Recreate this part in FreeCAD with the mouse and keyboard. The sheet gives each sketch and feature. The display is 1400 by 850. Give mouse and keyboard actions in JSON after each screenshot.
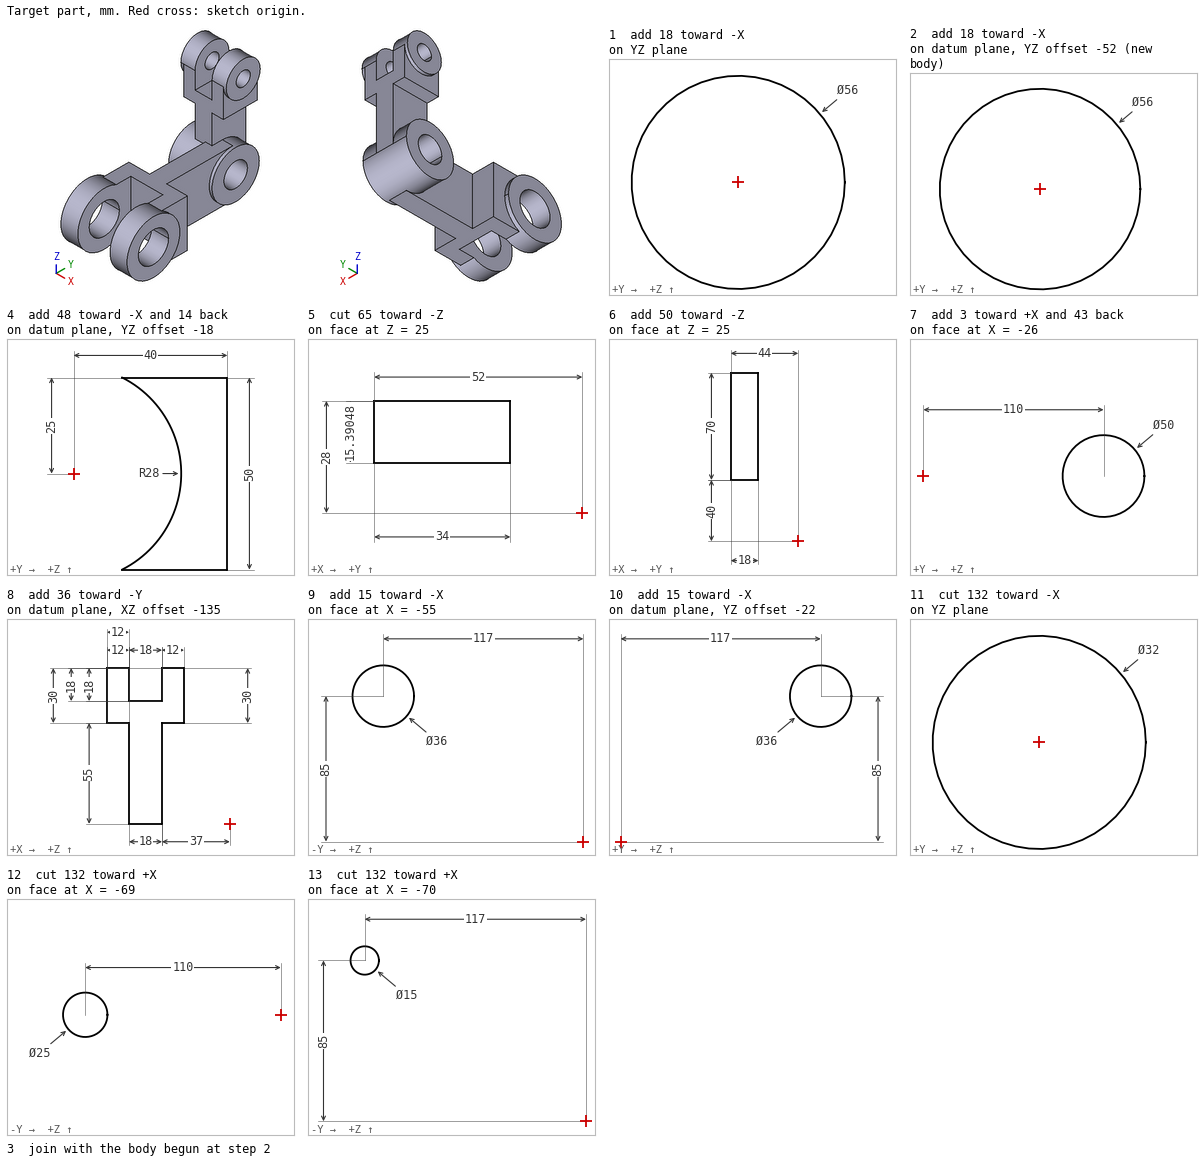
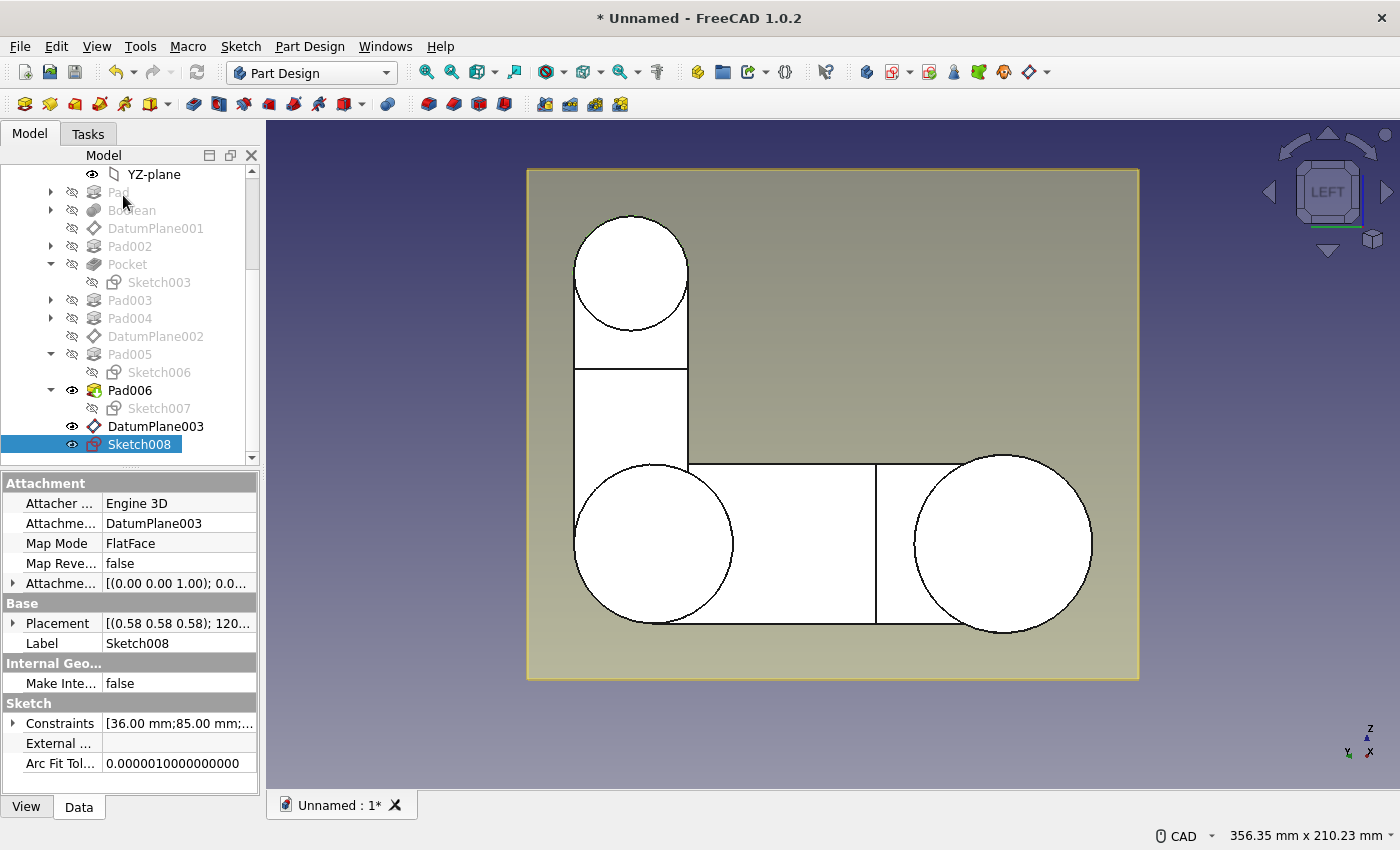
{"action": "left_click", "coordinate": [25, 104]}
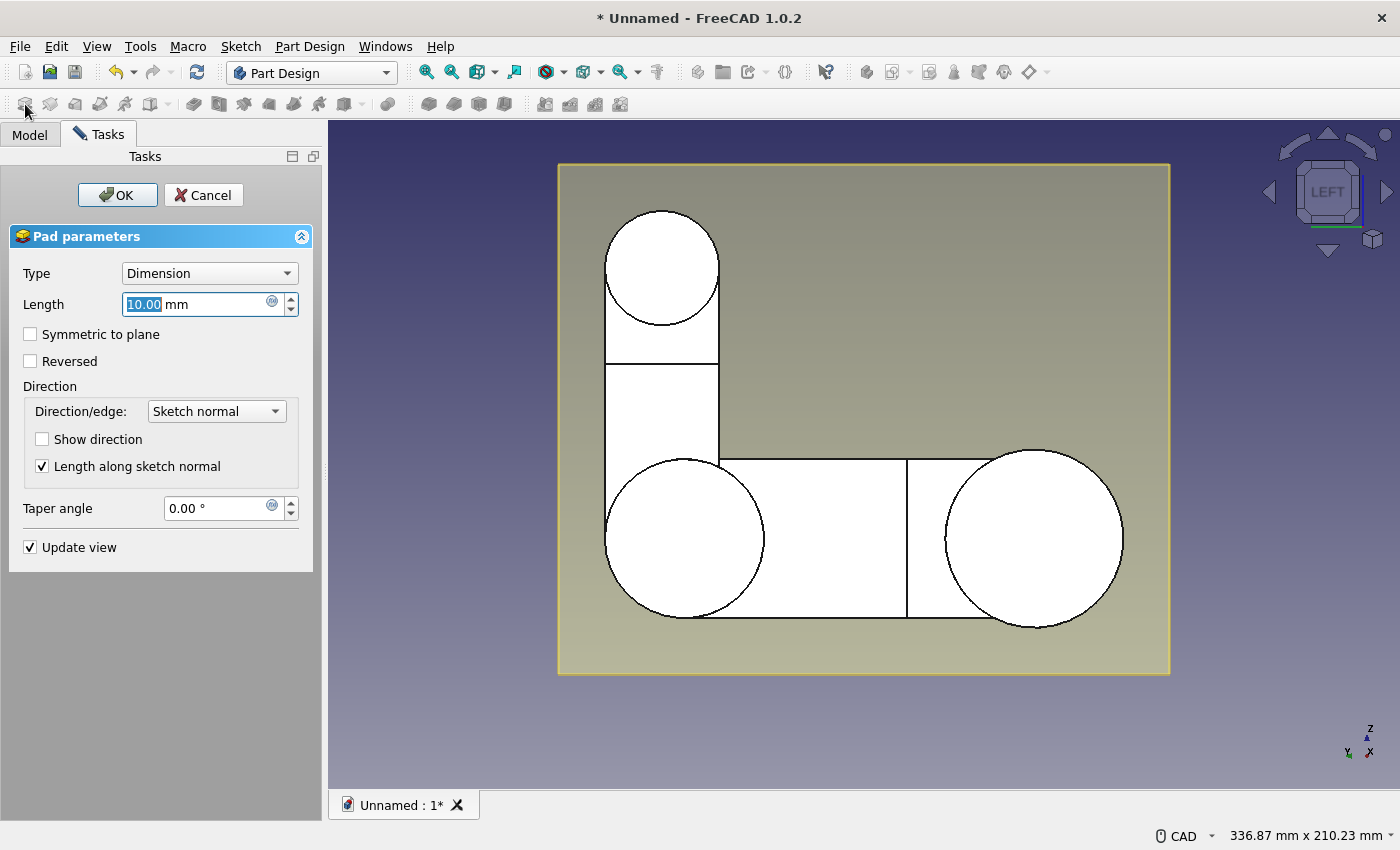
{"action": "type", "text": "15"}
{"action": "key", "text": "Tab"}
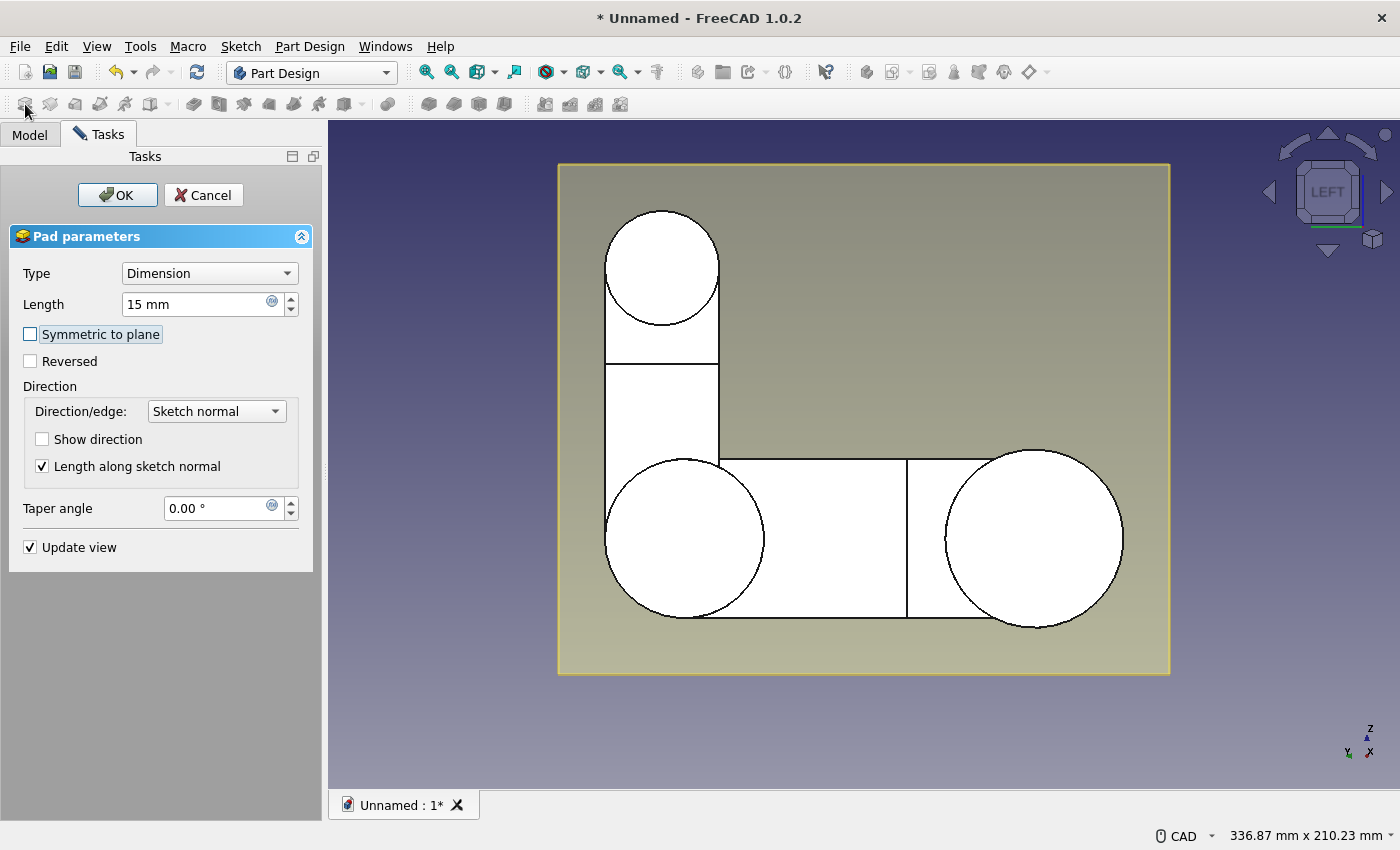
{"action": "left_click", "coordinate": [31, 361]}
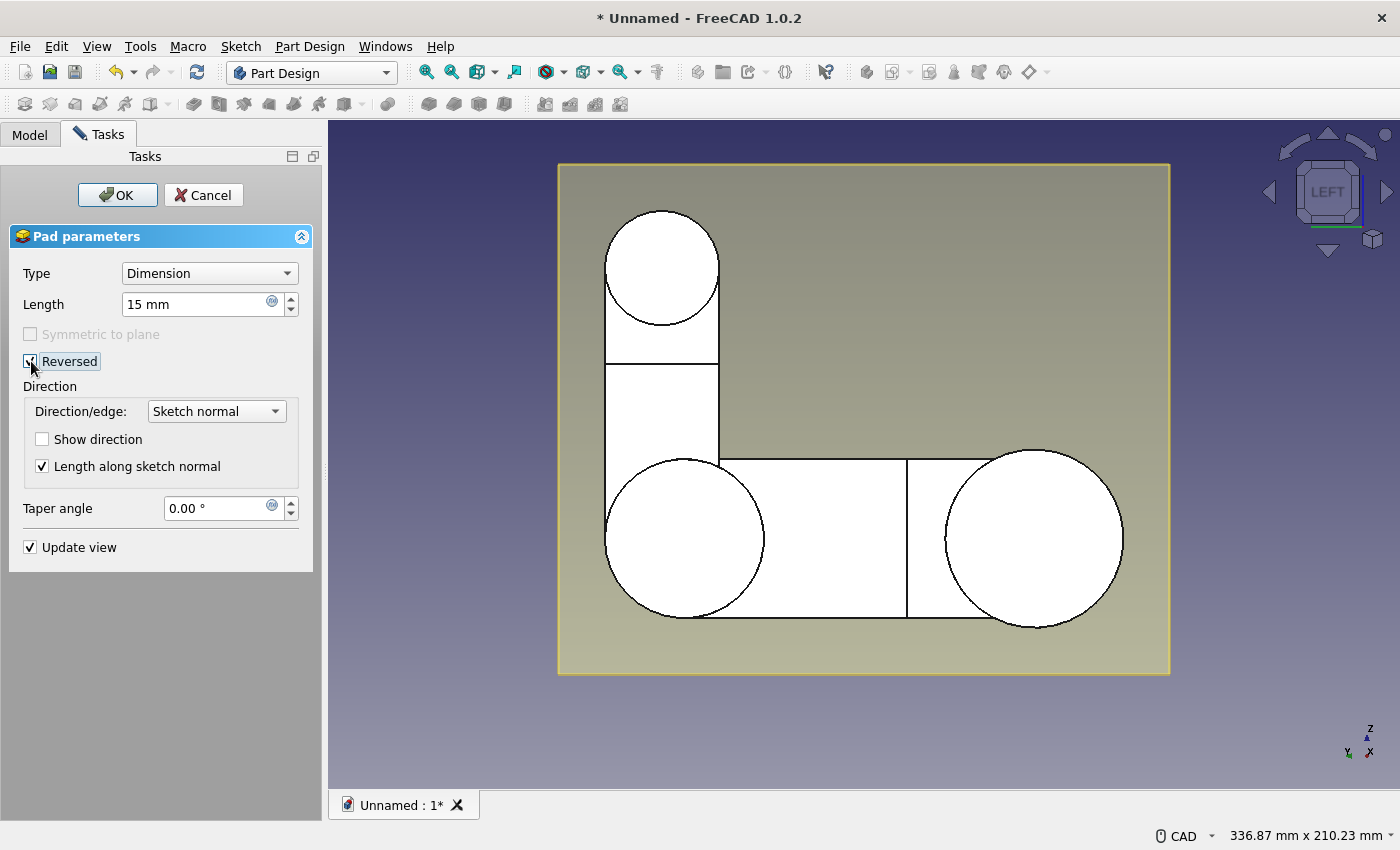
{"action": "left_click", "coordinate": [118, 195]}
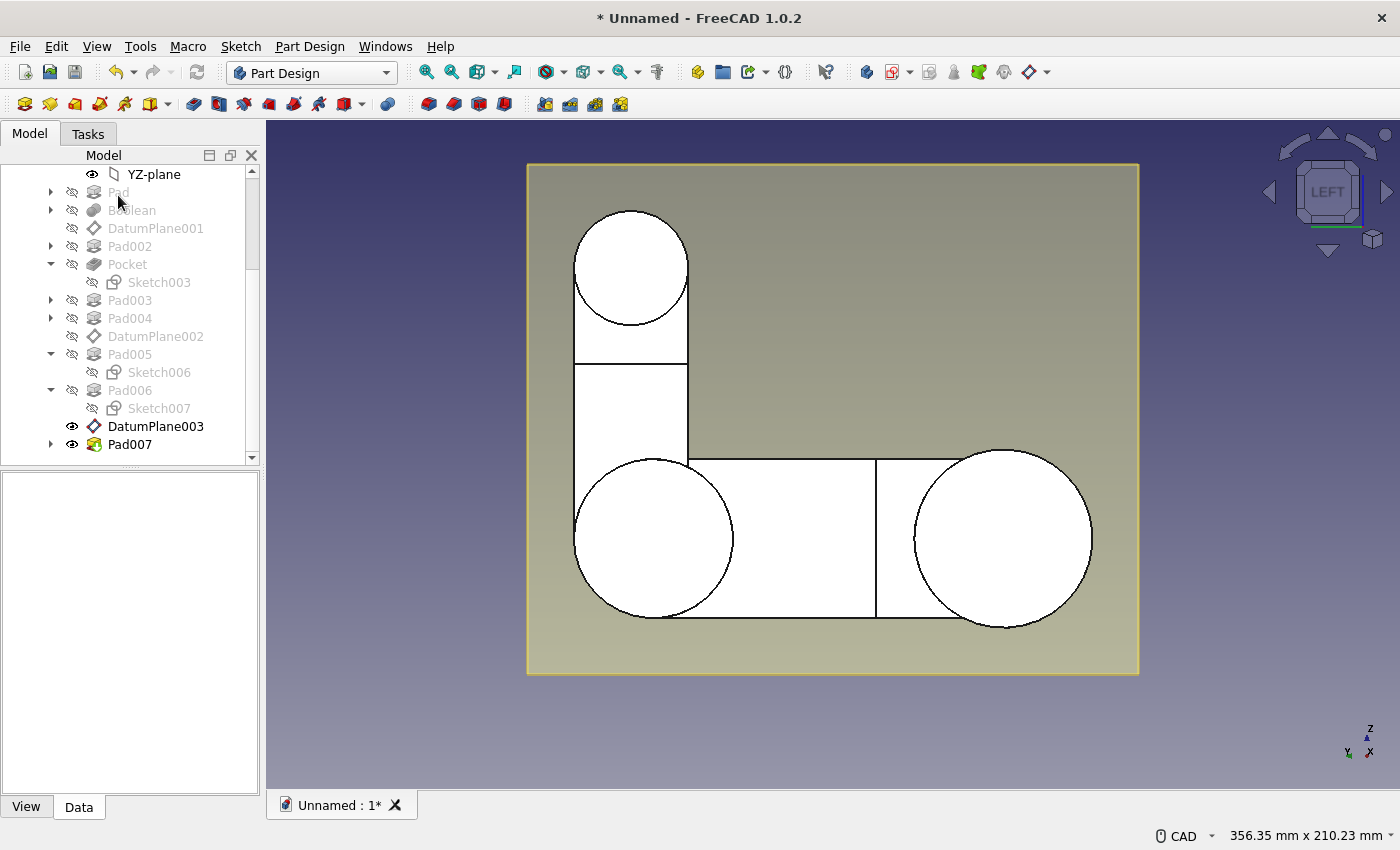
{"action": "left_click", "coordinate": [117, 426]}
{"action": "key", "text": "space"}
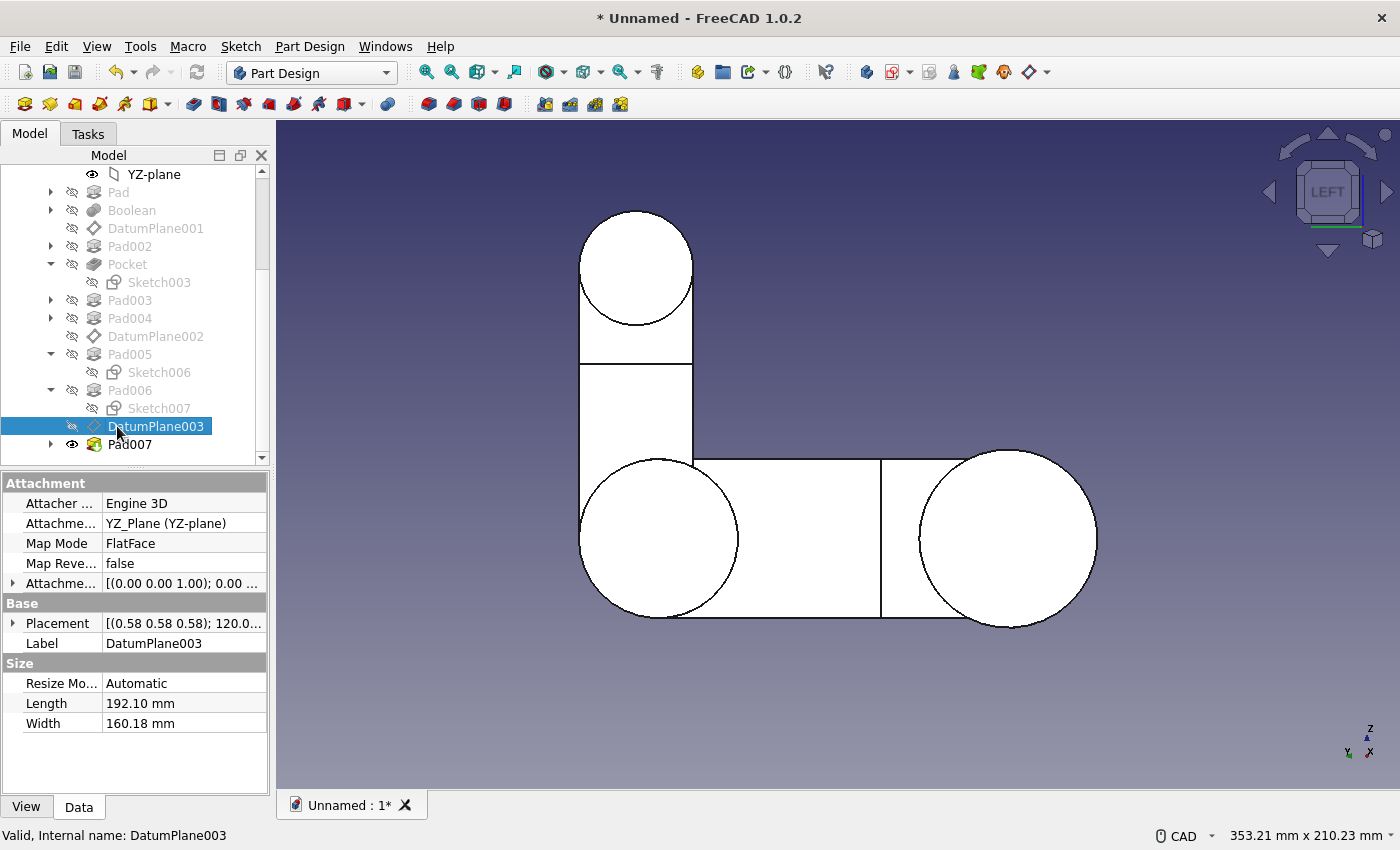
{"action": "left_click", "coordinate": [316, 749]}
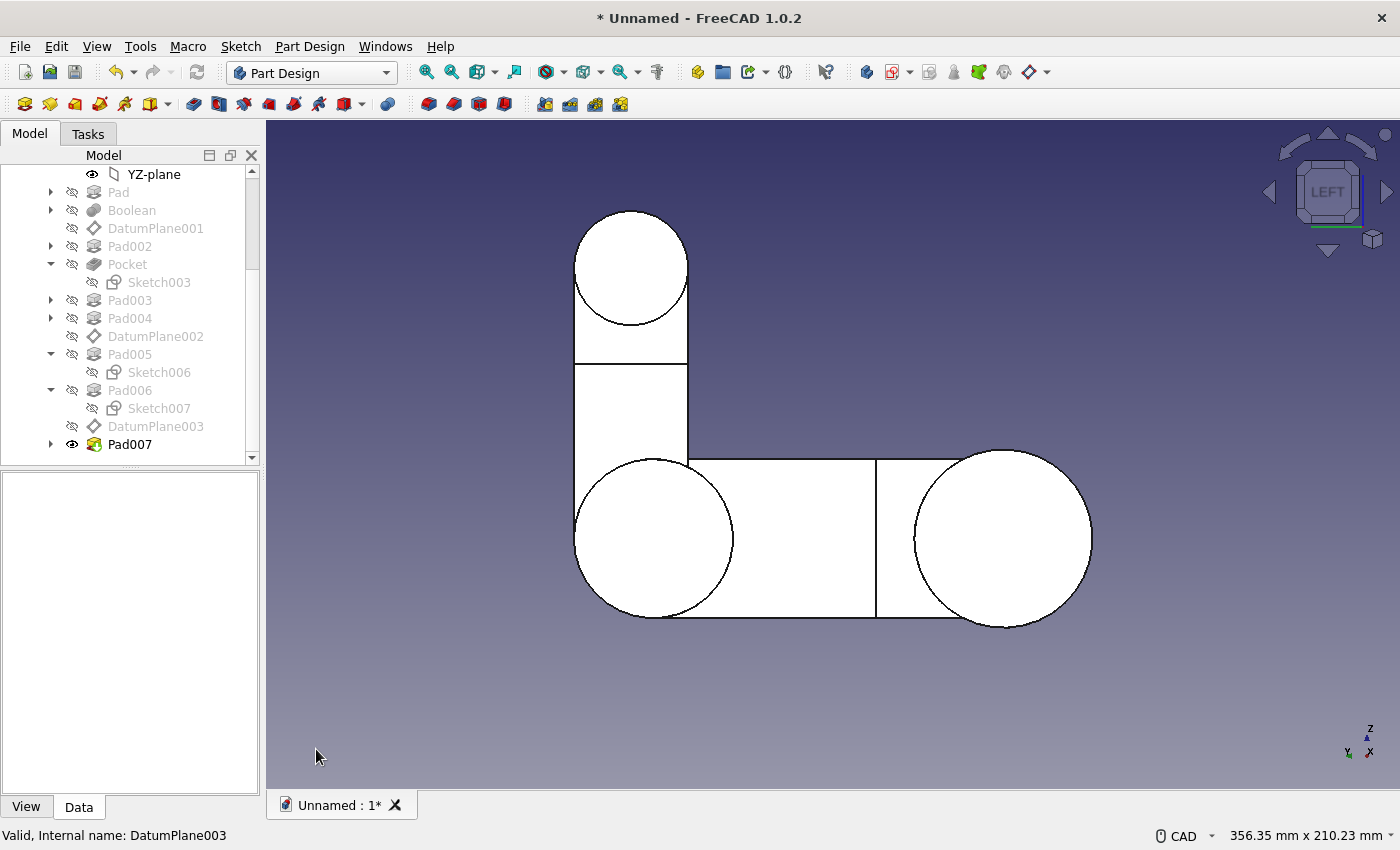
{"action": "left_click", "coordinate": [892, 72]}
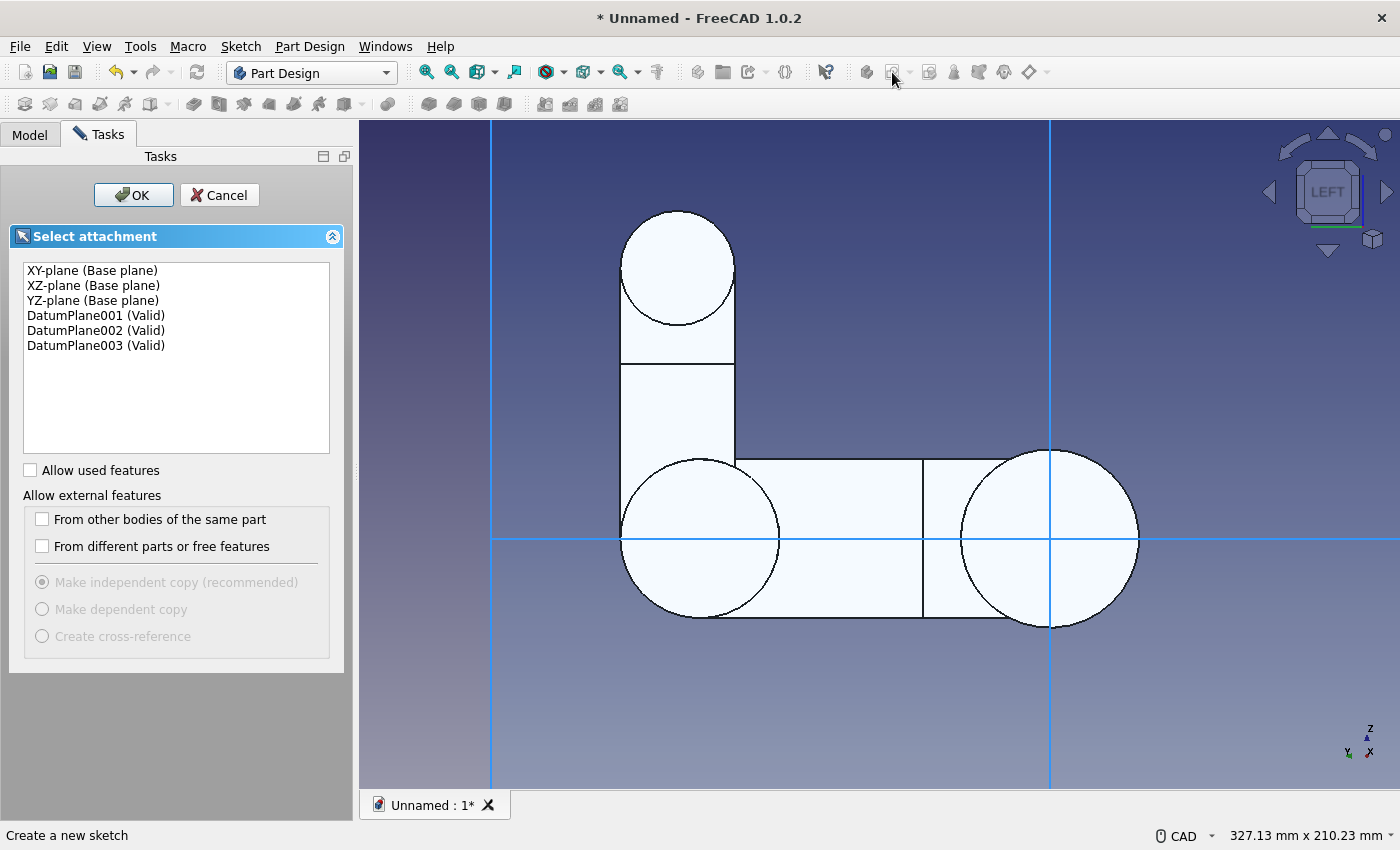
{"action": "left_click", "coordinate": [84, 300]}